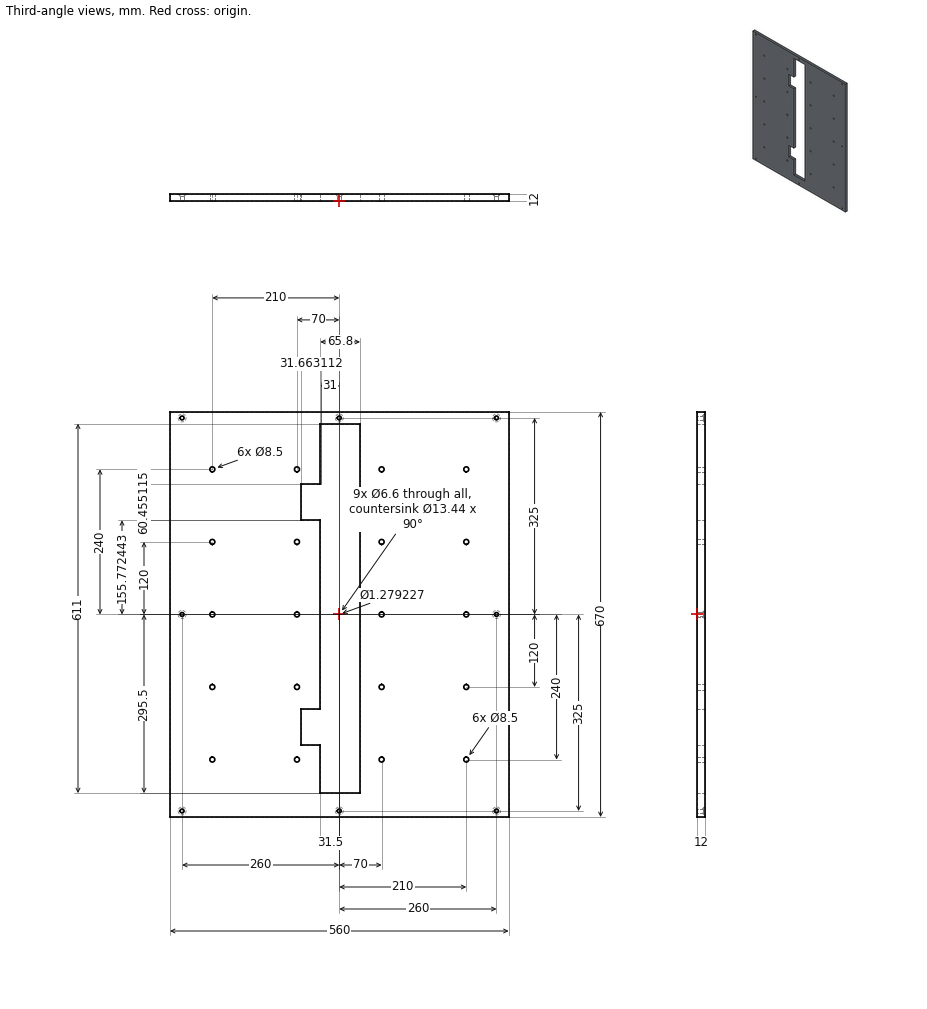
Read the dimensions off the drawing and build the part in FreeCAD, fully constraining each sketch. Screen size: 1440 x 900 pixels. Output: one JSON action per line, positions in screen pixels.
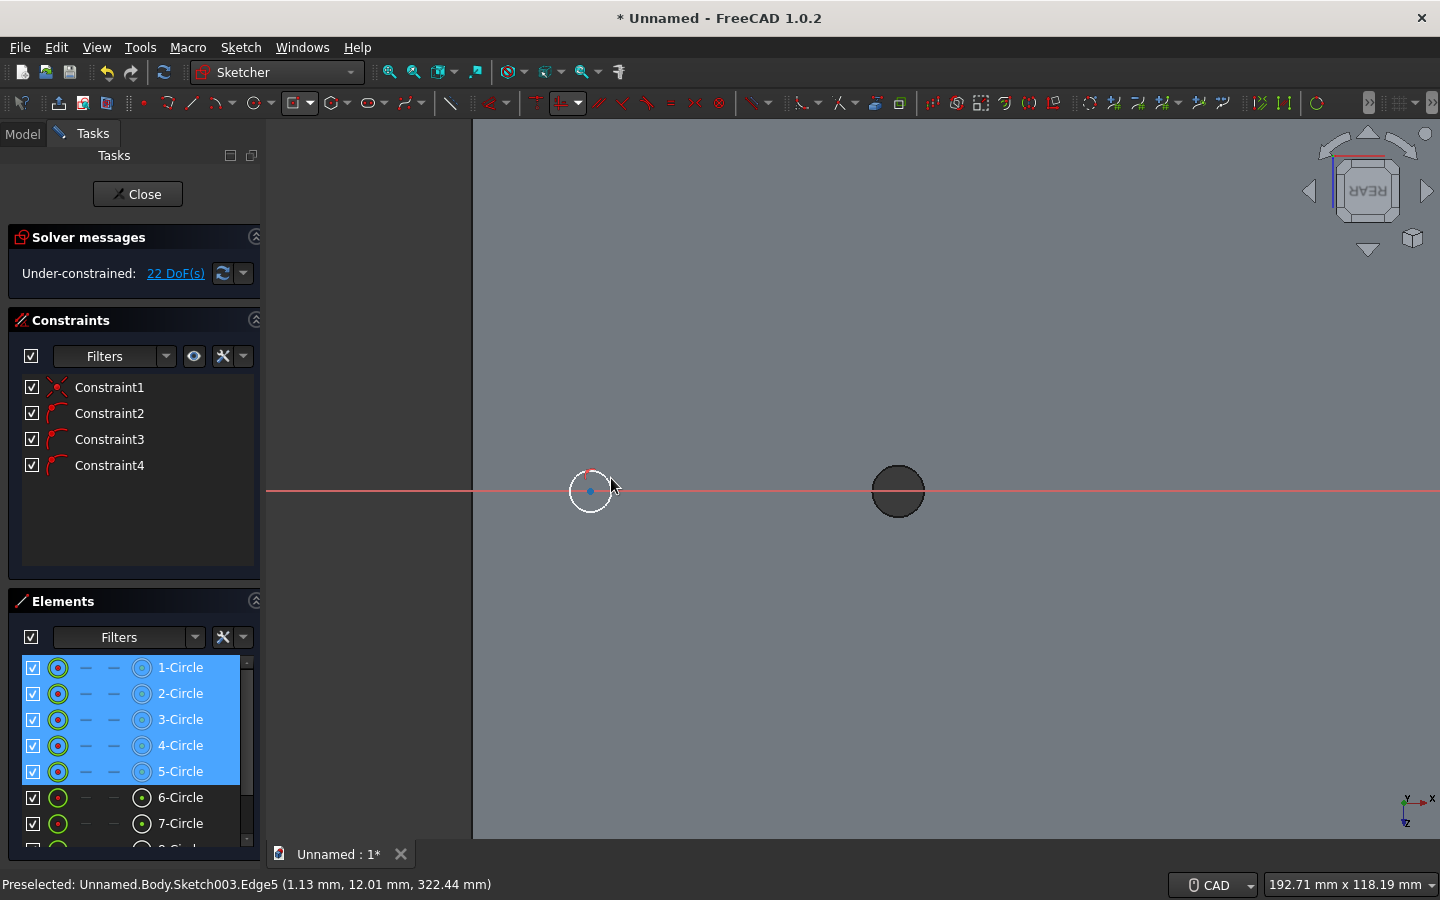
{"action": "left_click", "coordinate": [605, 477]}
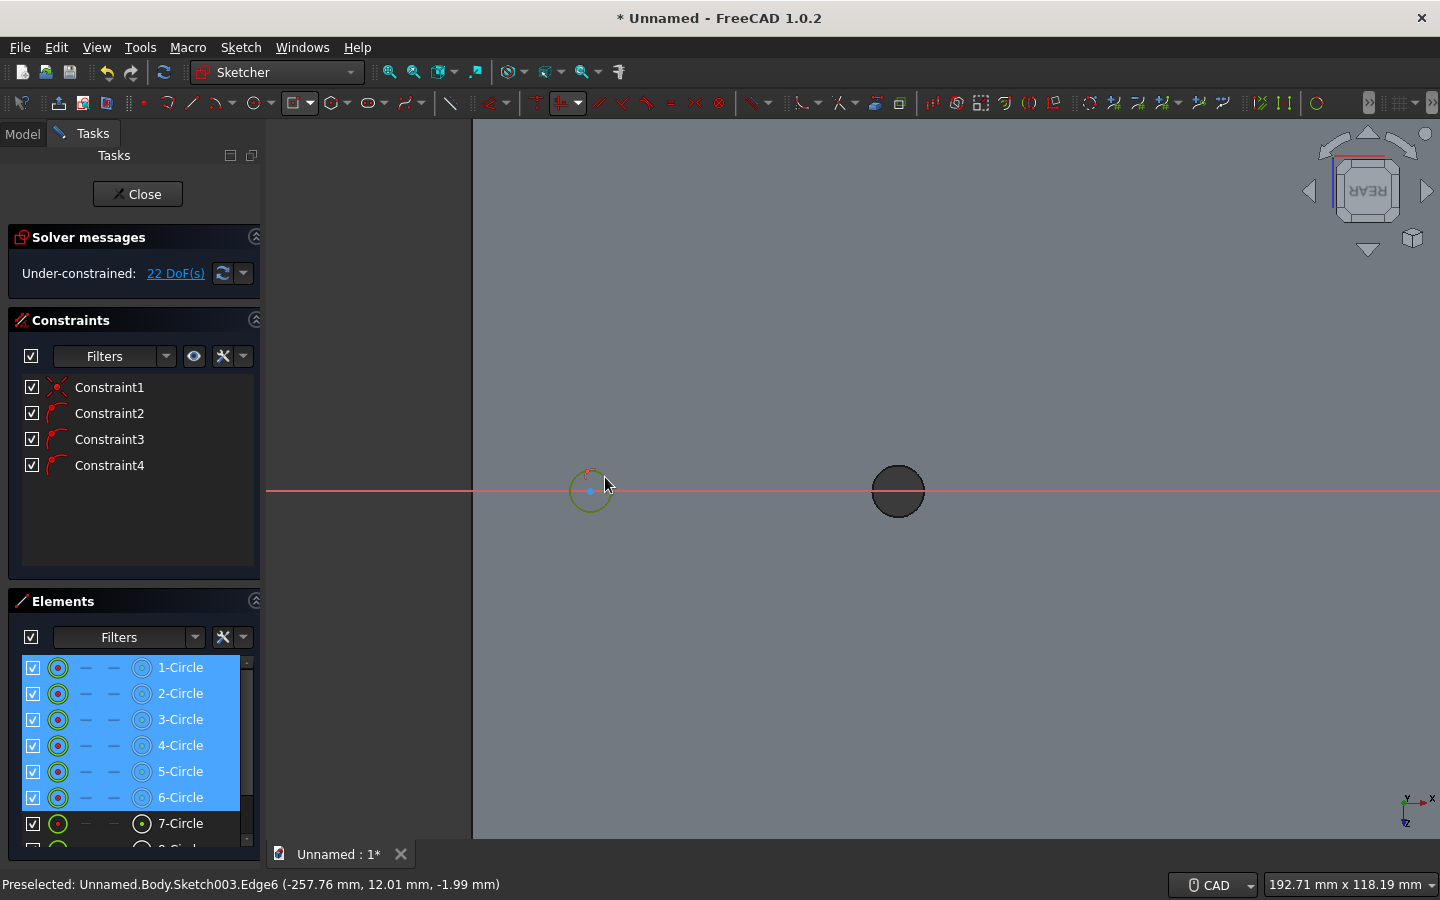
{"action": "scroll", "coordinate": [611, 477], "scroll_direction": "down", "scroll_amount": 11}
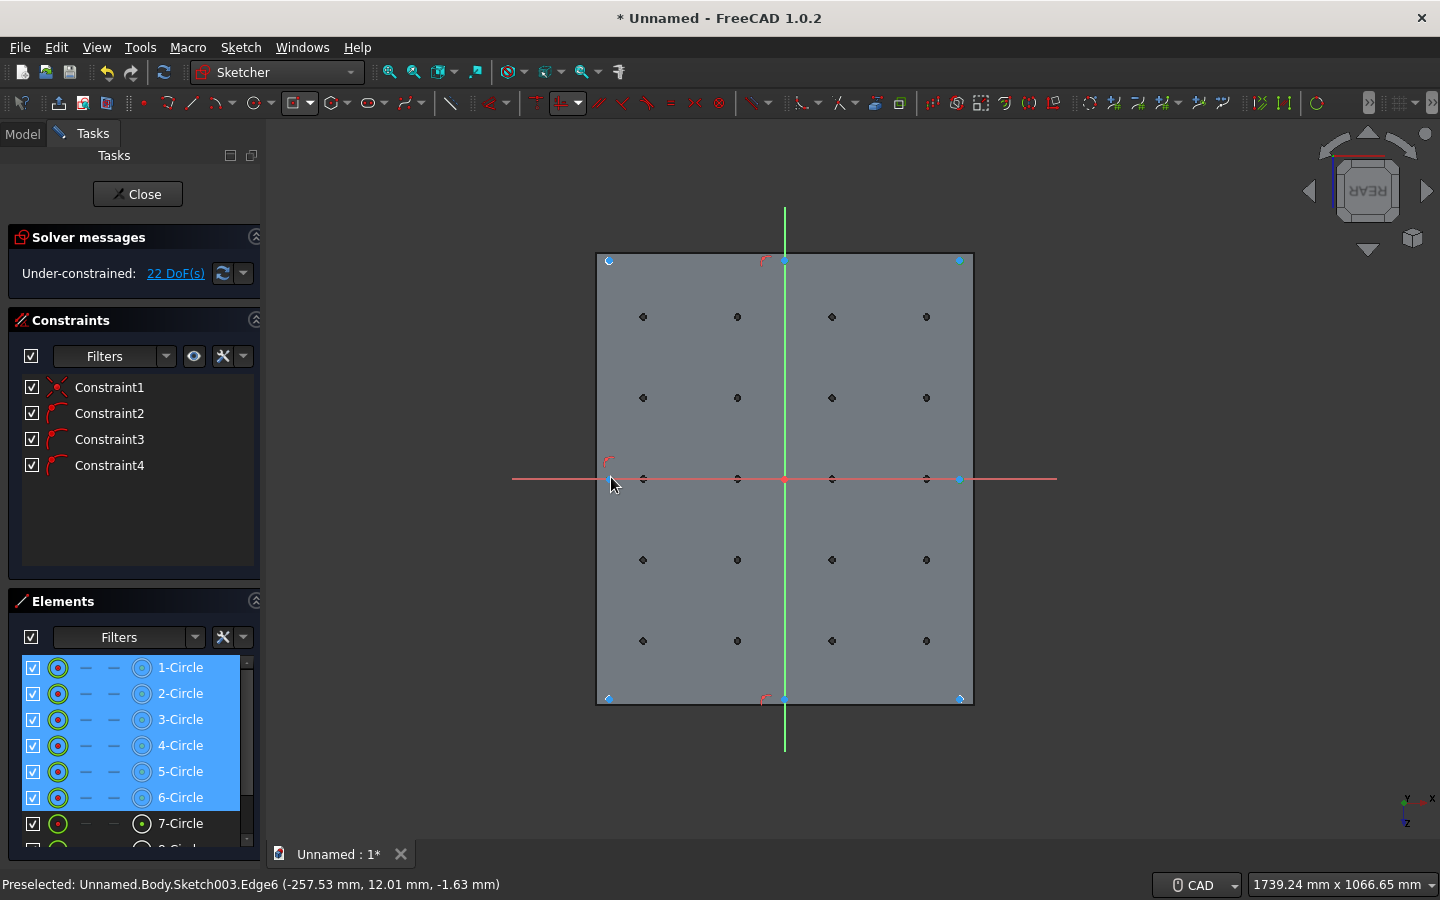
{"action": "scroll", "coordinate": [611, 259], "scroll_direction": "up", "scroll_amount": 8}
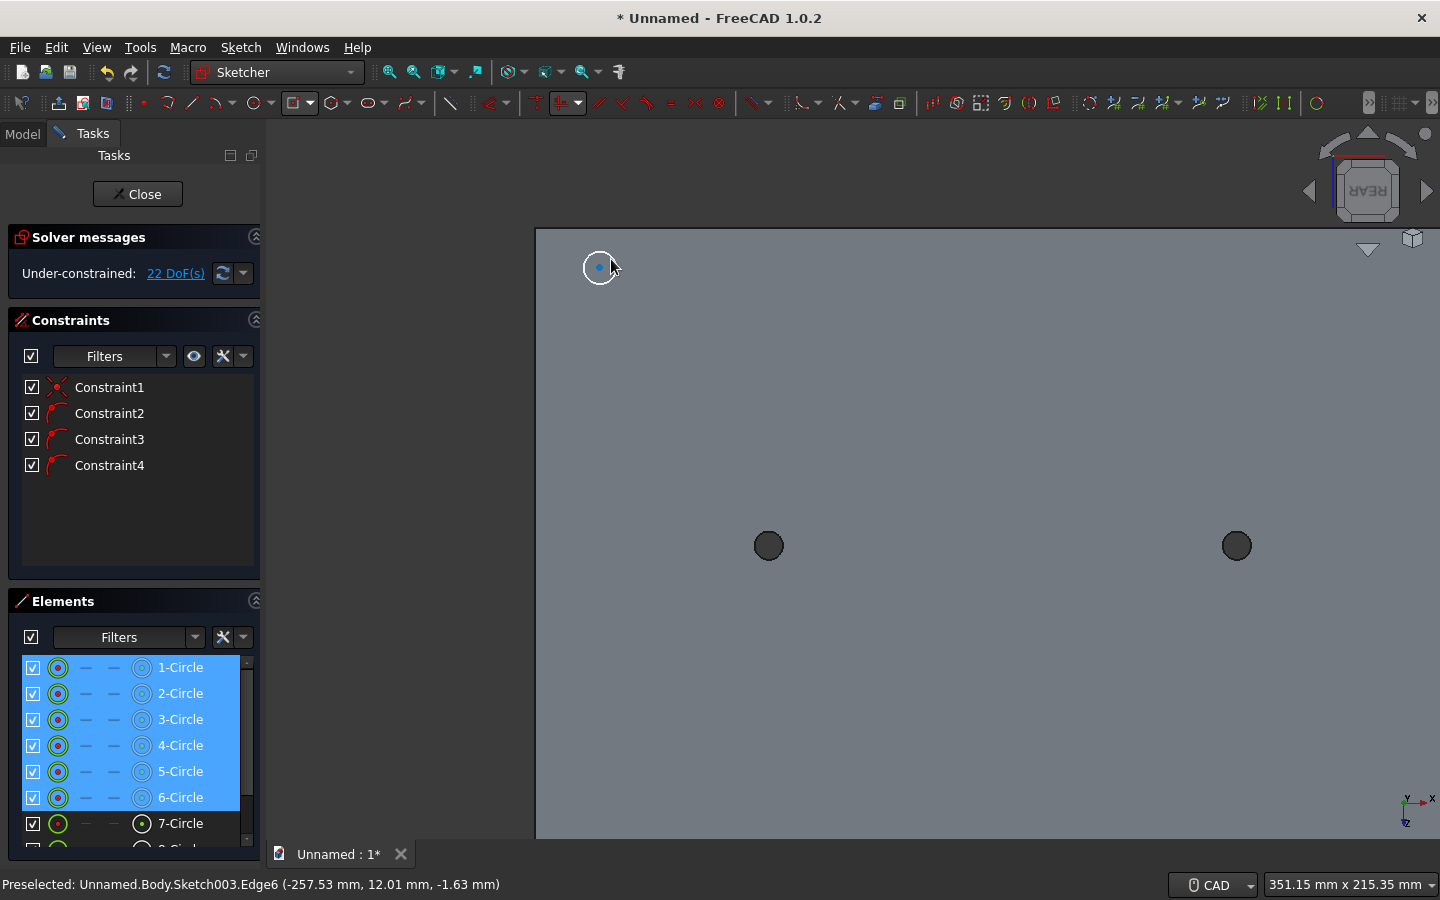
{"action": "left_click", "coordinate": [611, 256]}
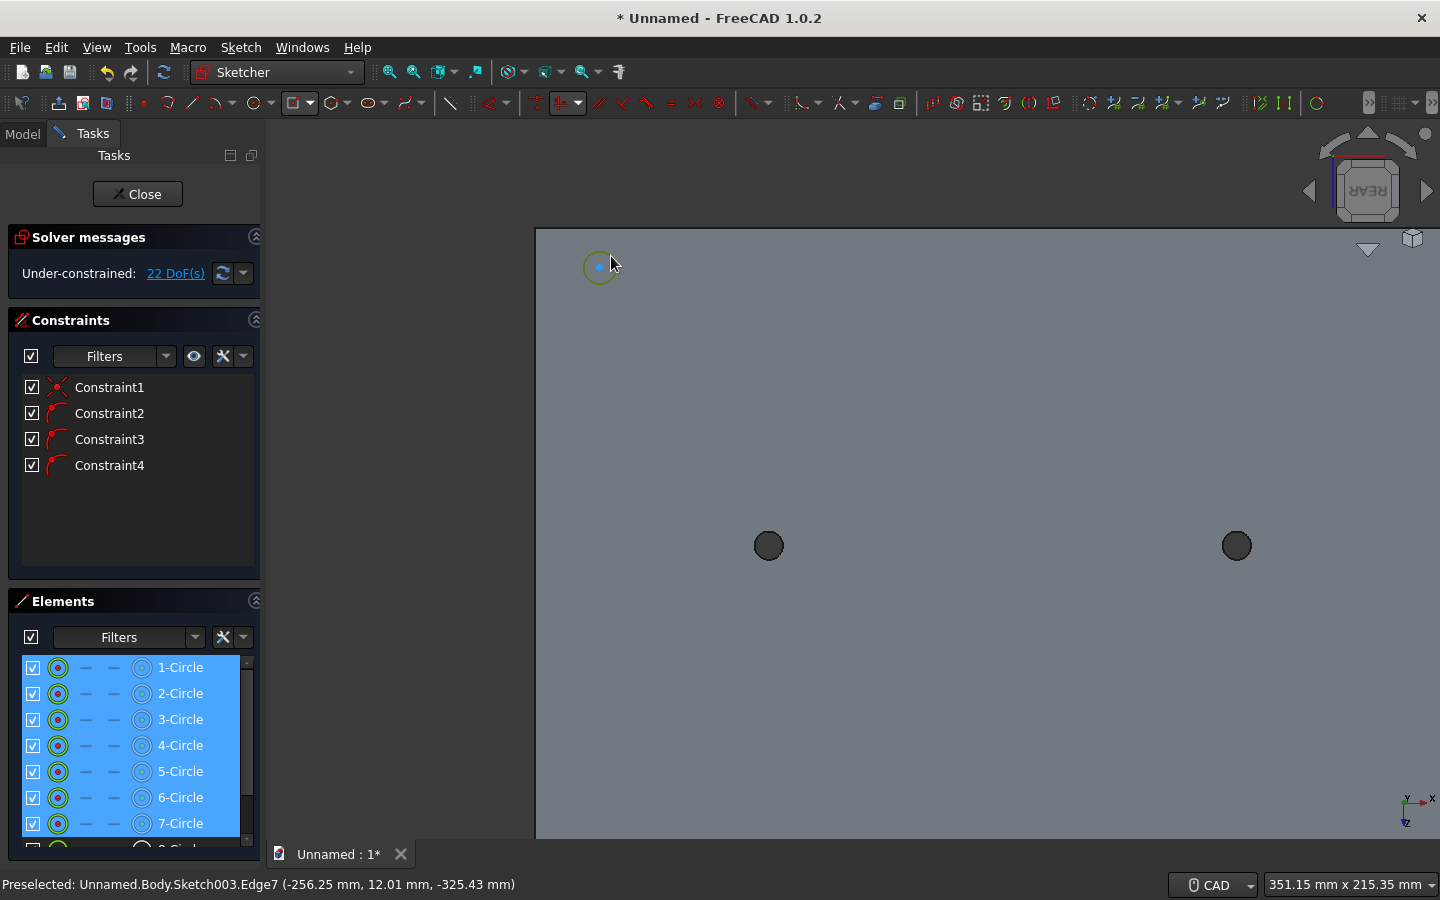
{"action": "scroll", "coordinate": [611, 259], "scroll_direction": "down", "scroll_amount": 8}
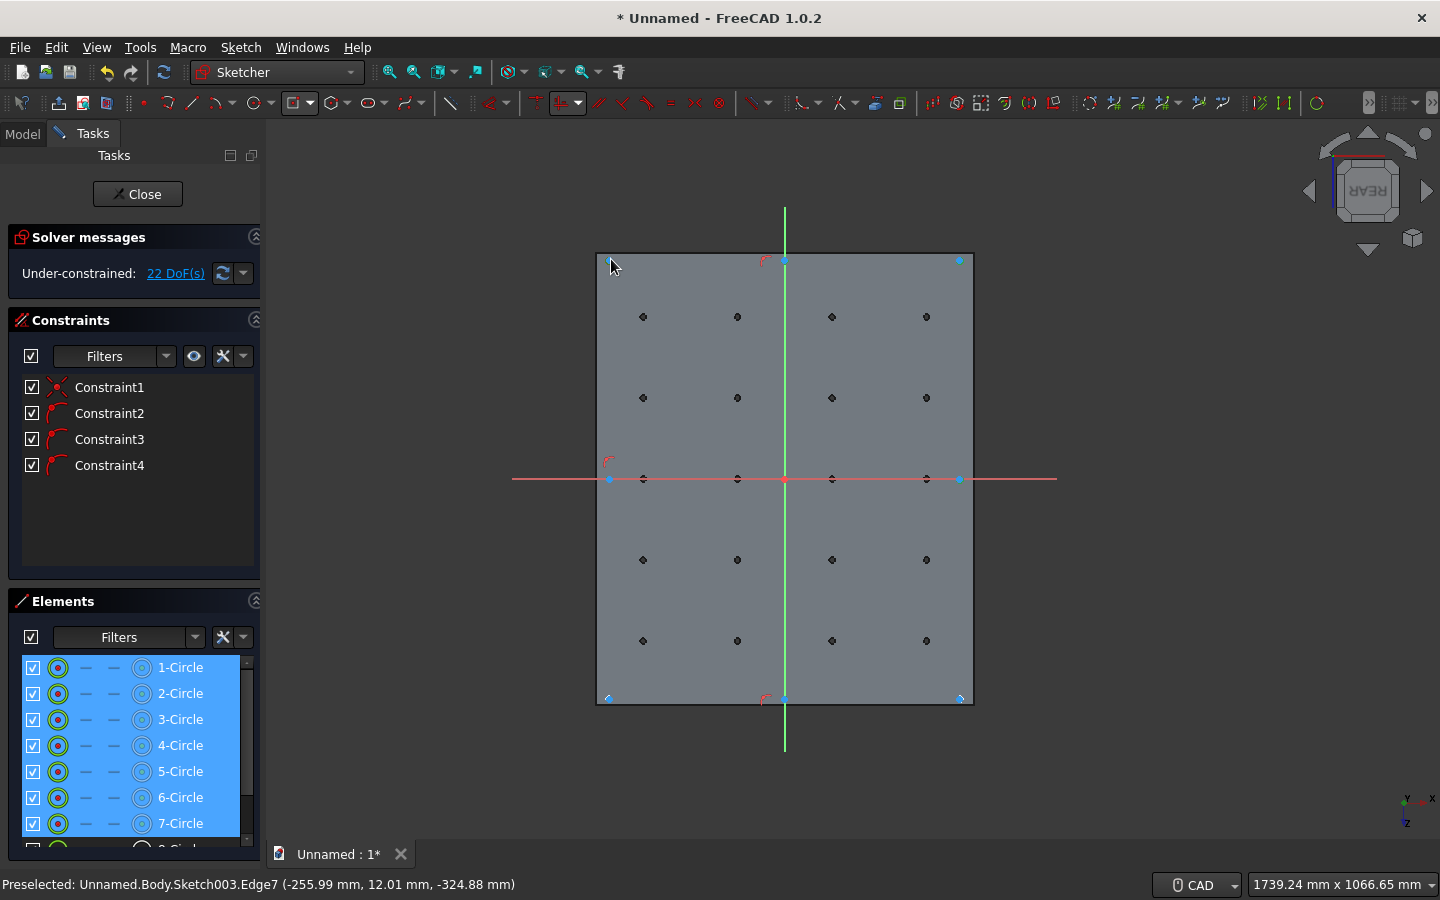
{"action": "scroll", "coordinate": [611, 697], "scroll_direction": "up", "scroll_amount": 8}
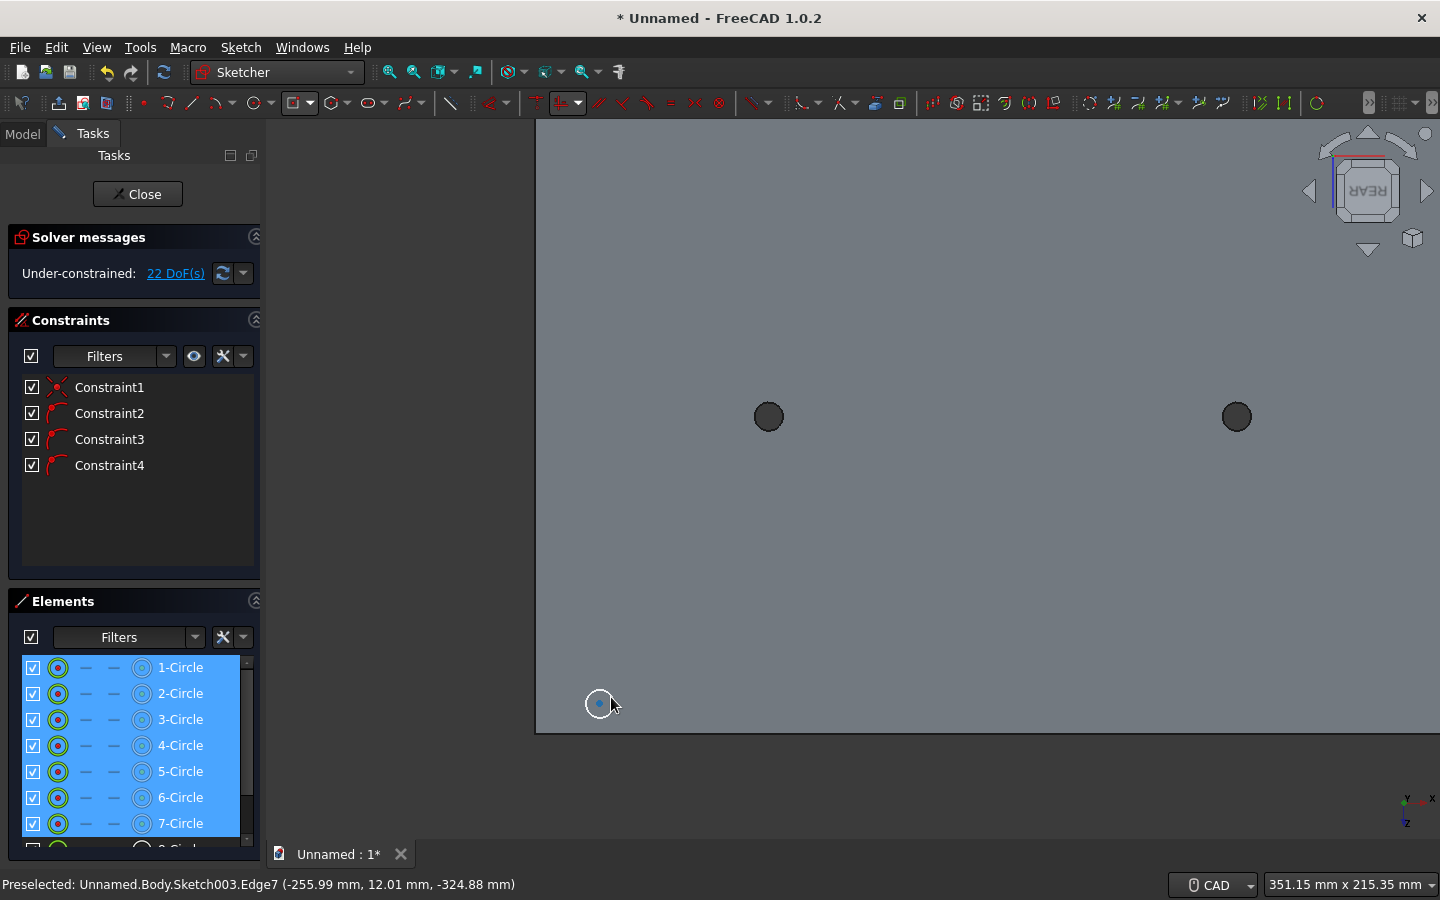
{"action": "left_click", "coordinate": [610, 694]}